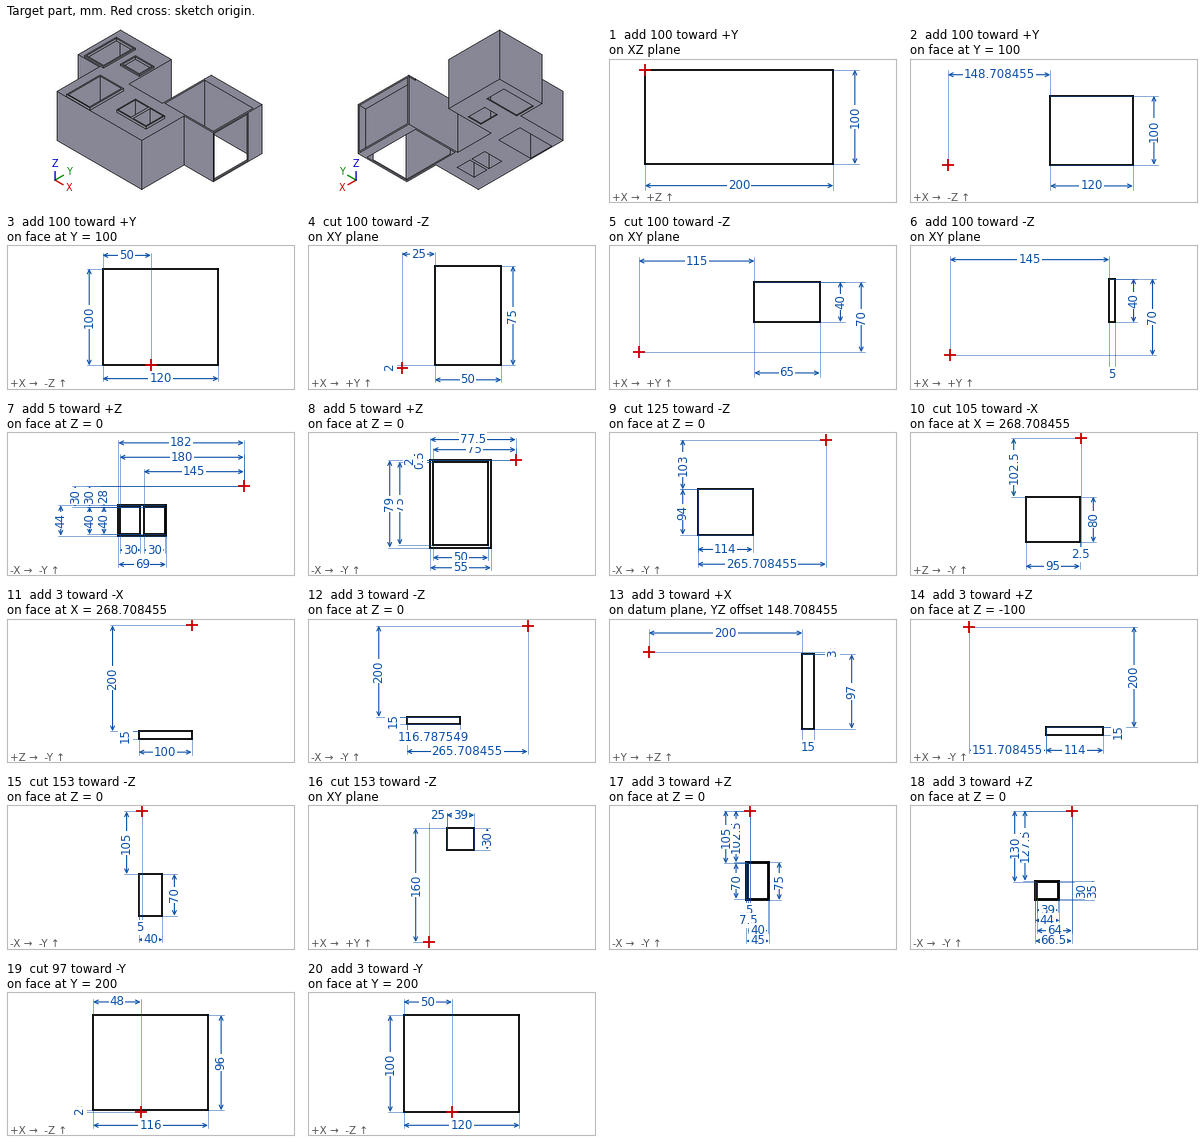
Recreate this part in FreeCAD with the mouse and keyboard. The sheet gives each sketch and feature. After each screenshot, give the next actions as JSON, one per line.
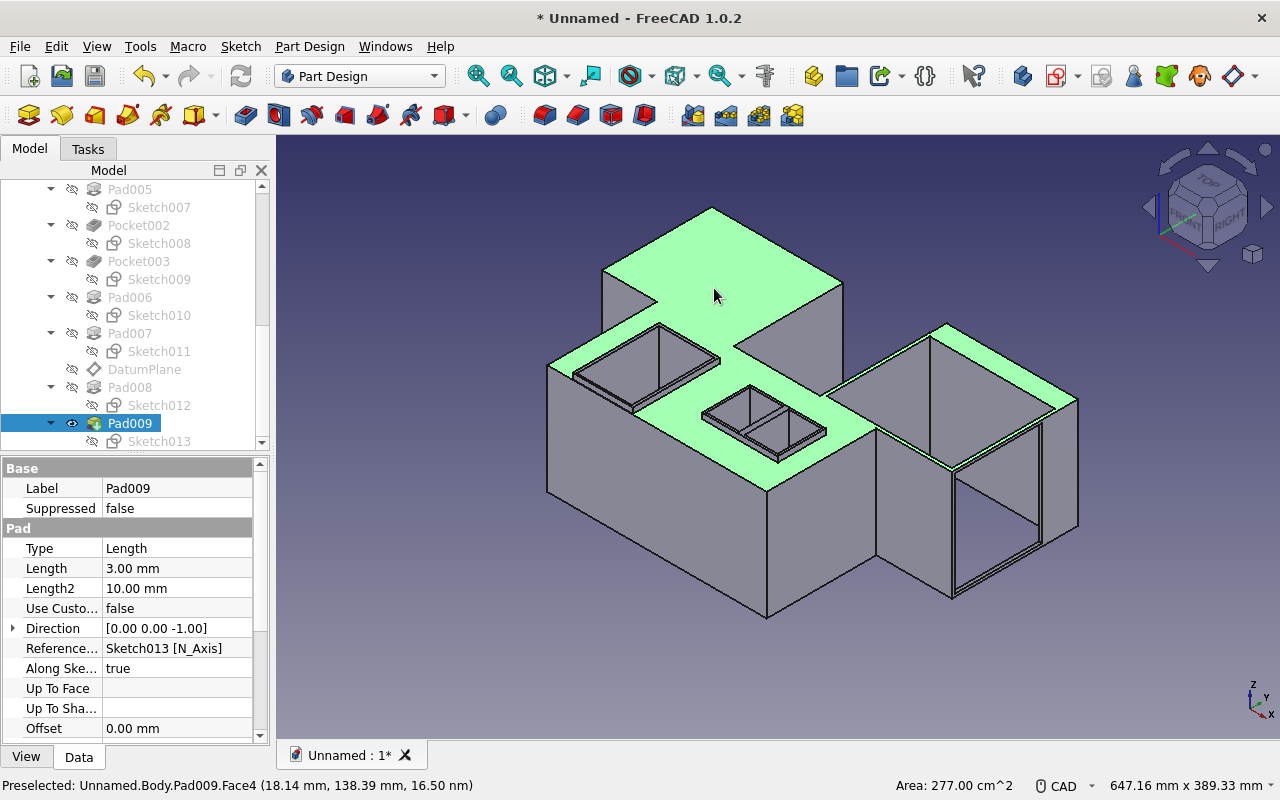
{"action": "left_click", "coordinate": [1056, 76]}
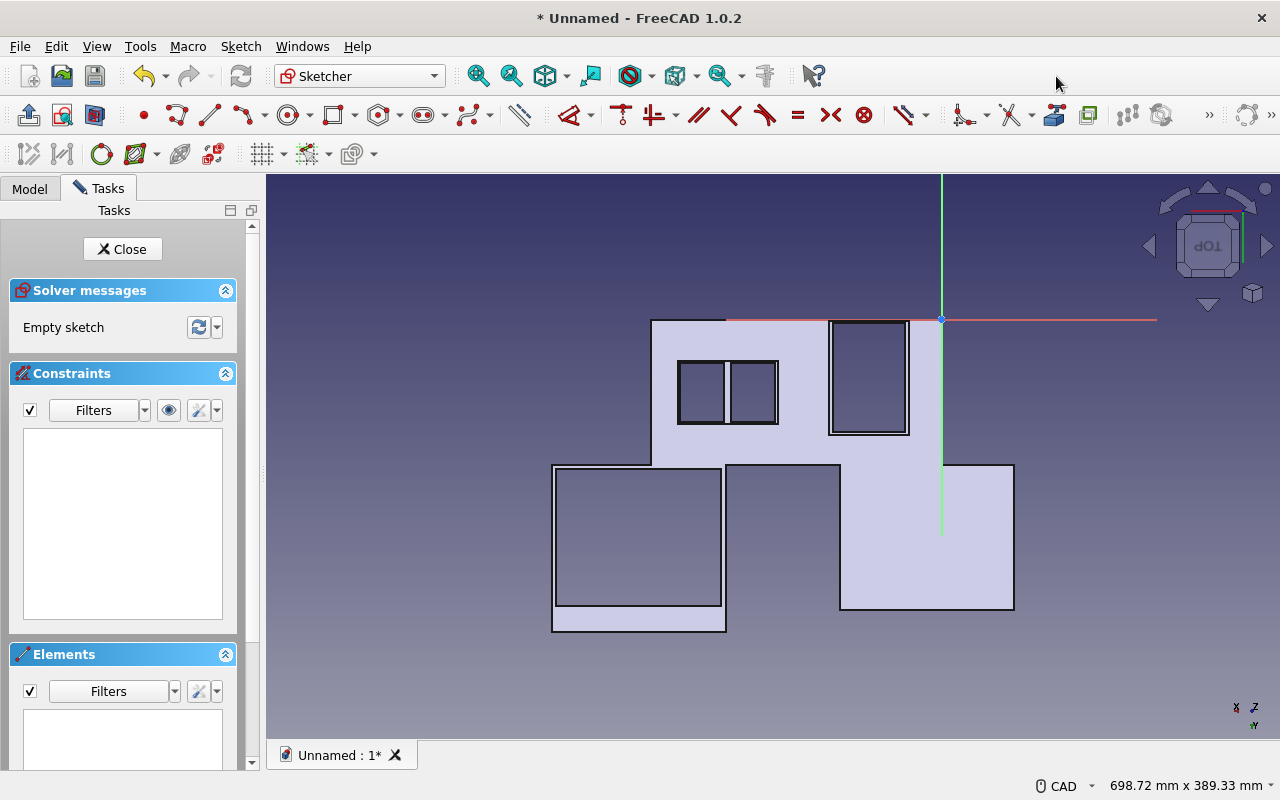
{"action": "left_click", "coordinate": [95, 116]}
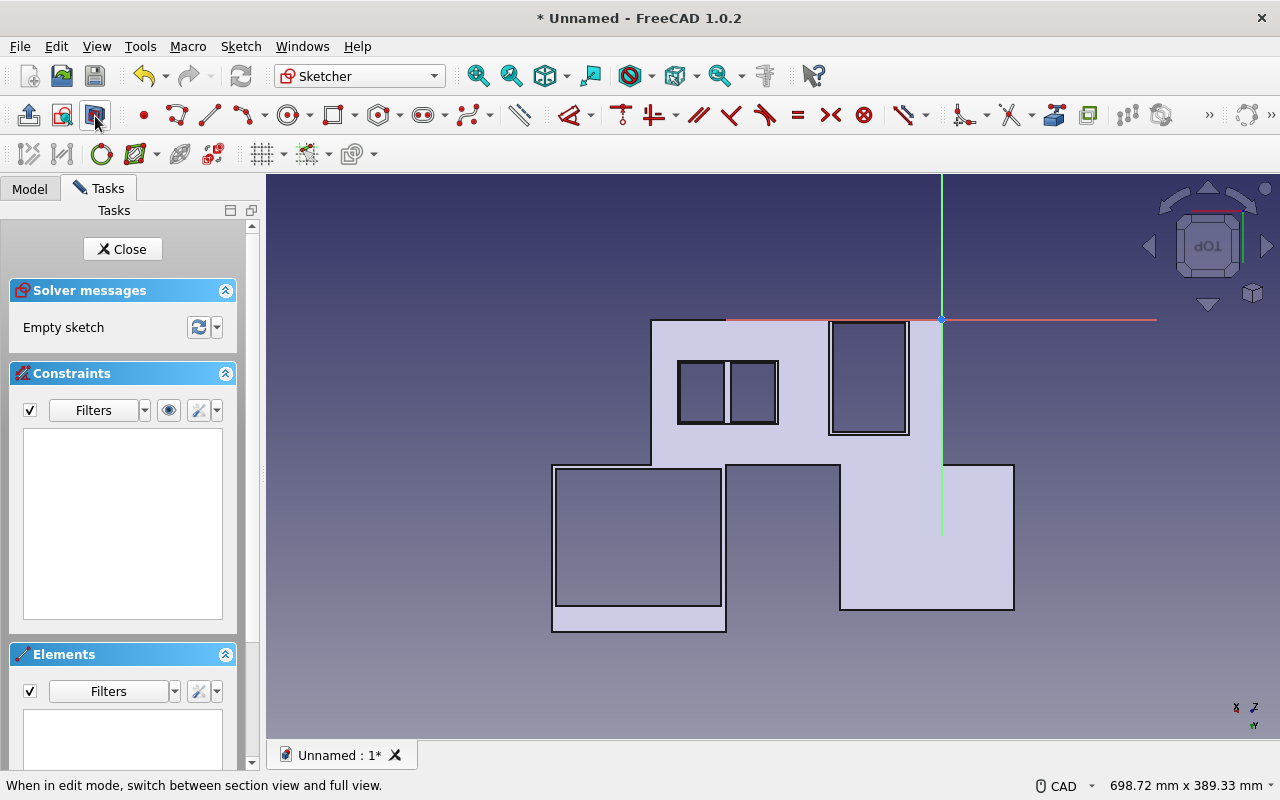
{"action": "scroll", "coordinate": [1075, 552], "scroll_direction": "up", "scroll_amount": 6}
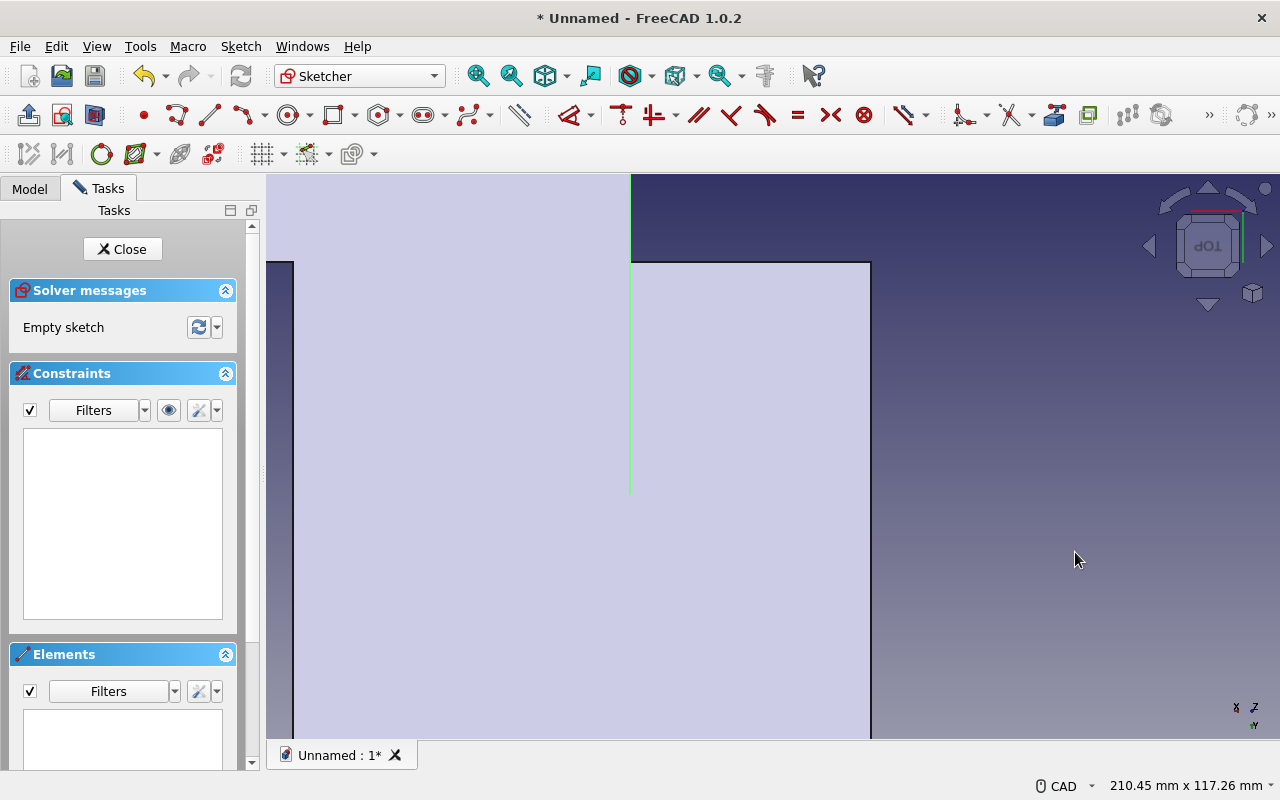
{"action": "left_click", "coordinate": [332, 116]}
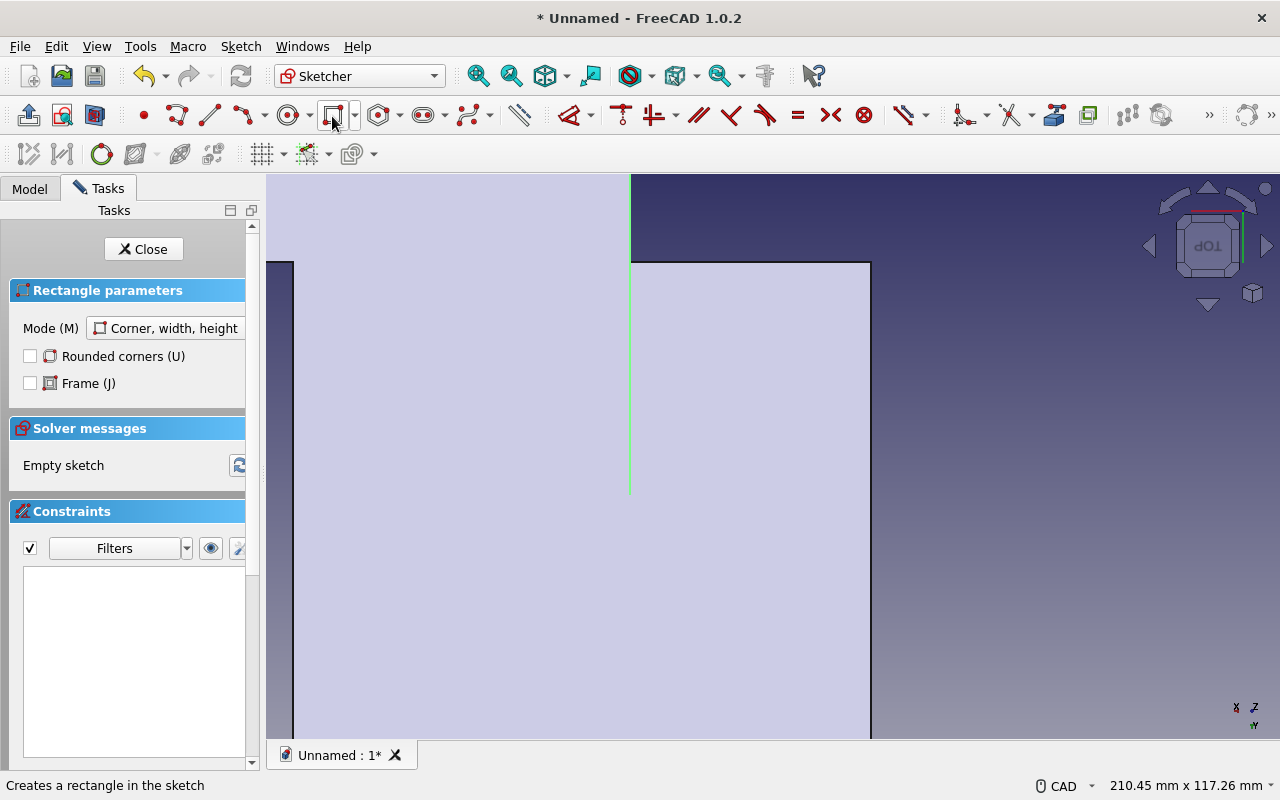
{"action": "left_click", "coordinate": [606, 286]}
{"action": "mouse_move", "coordinate": [799, 623]}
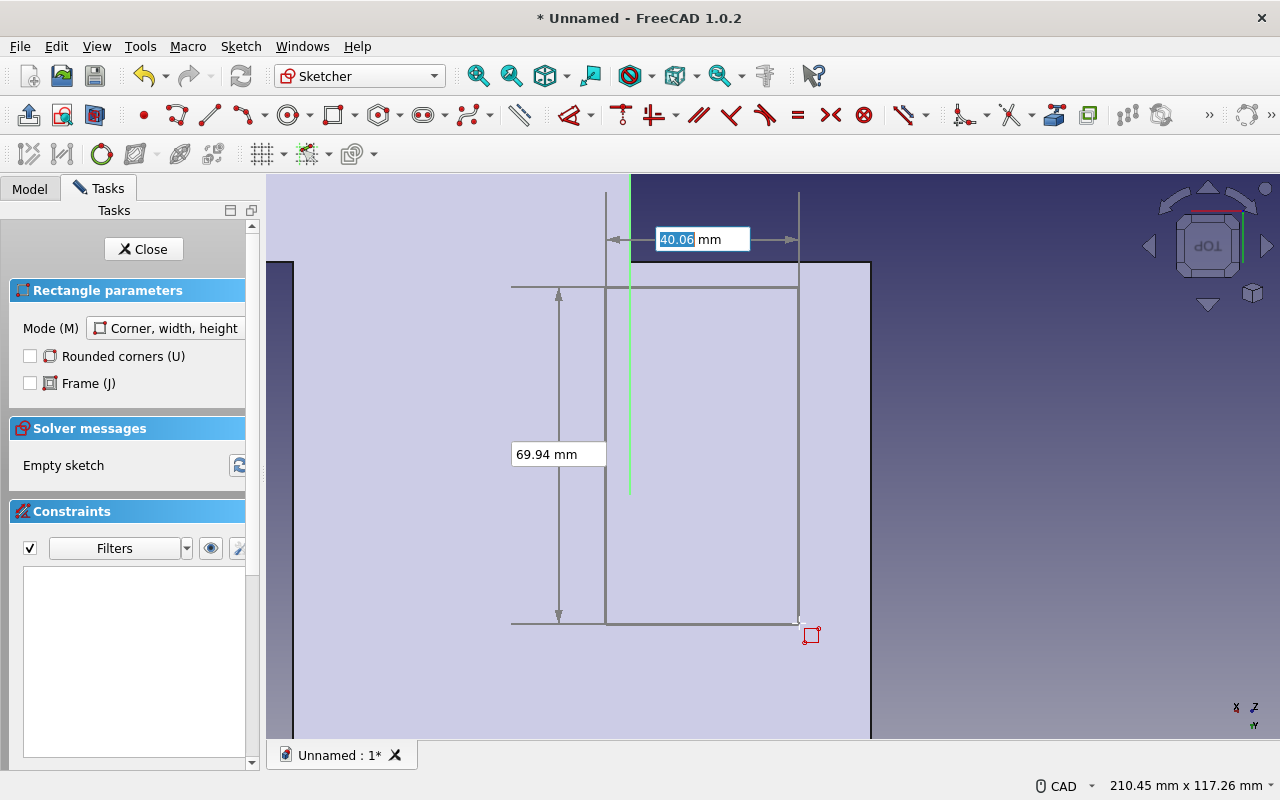
{"action": "type", "text": "40"}
{"action": "key", "text": "Tab"}
{"action": "type", "text": "70"}
{"action": "key", "text": "Return"}
{"action": "key", "text": "Escape"}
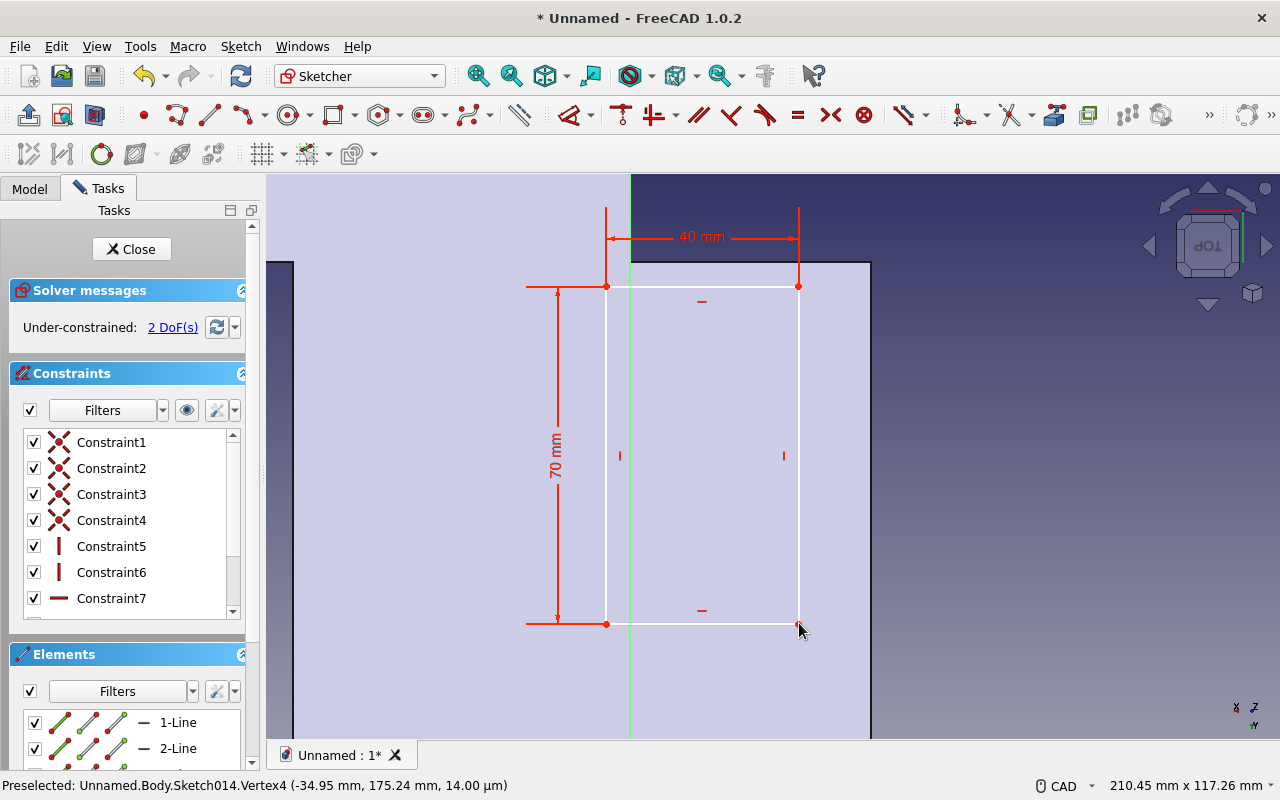
{"action": "left_click", "coordinate": [568, 116]}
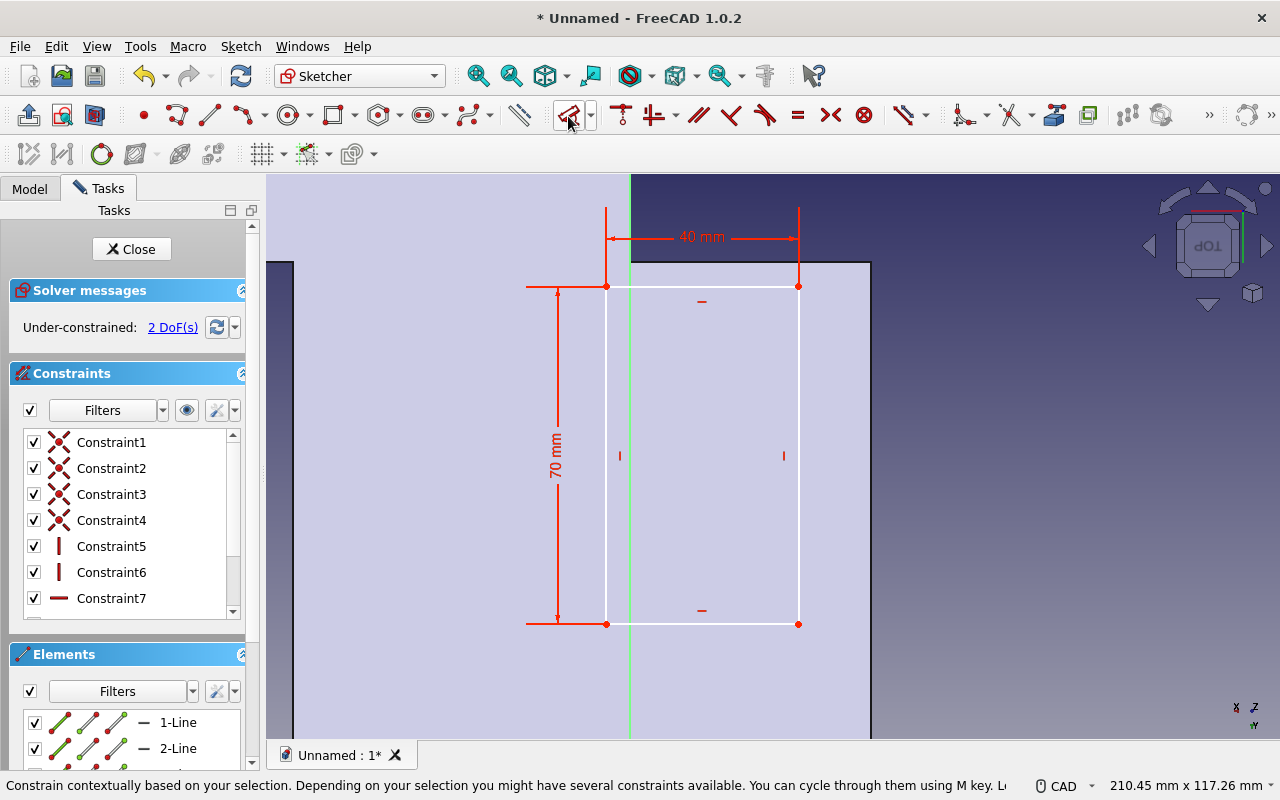
{"action": "scroll", "coordinate": [606, 287], "scroll_direction": "up", "scroll_amount": 3}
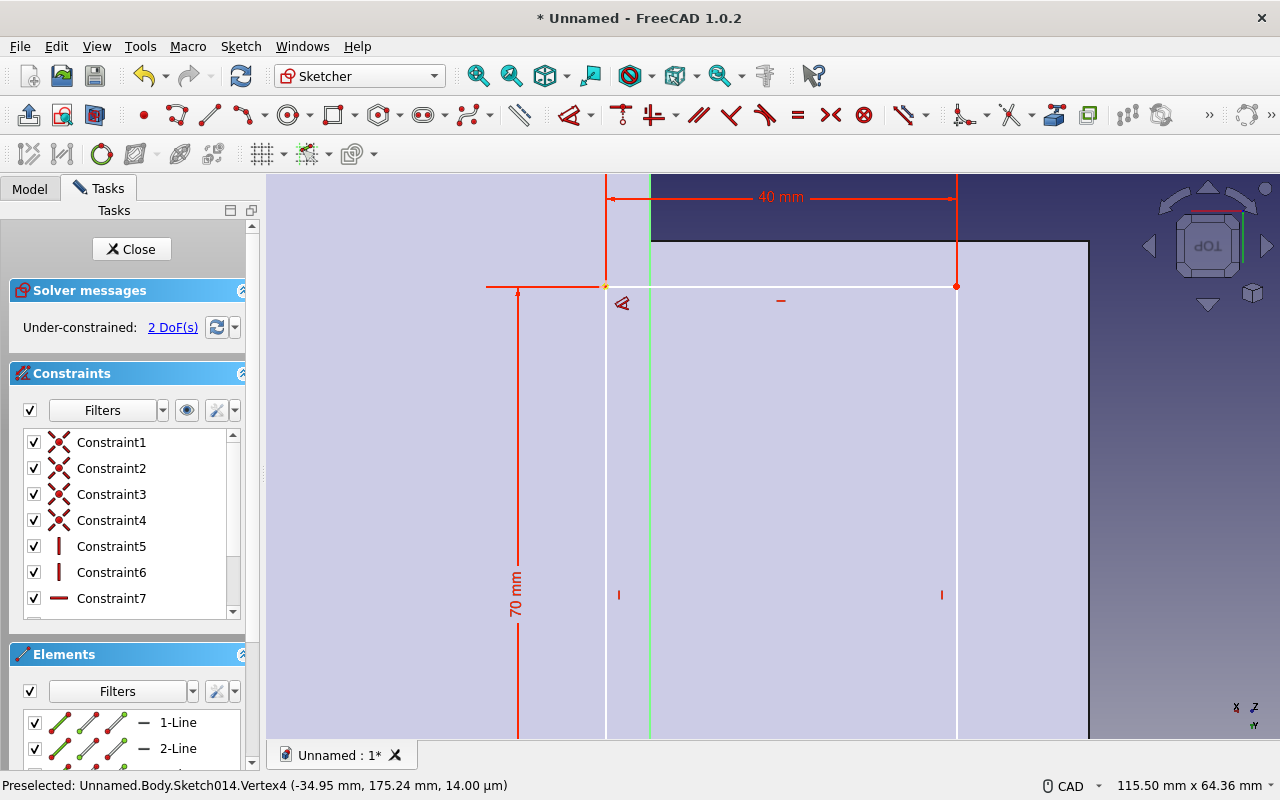
{"action": "left_click", "coordinate": [606, 287]}
{"action": "left_click", "coordinate": [628, 321]}